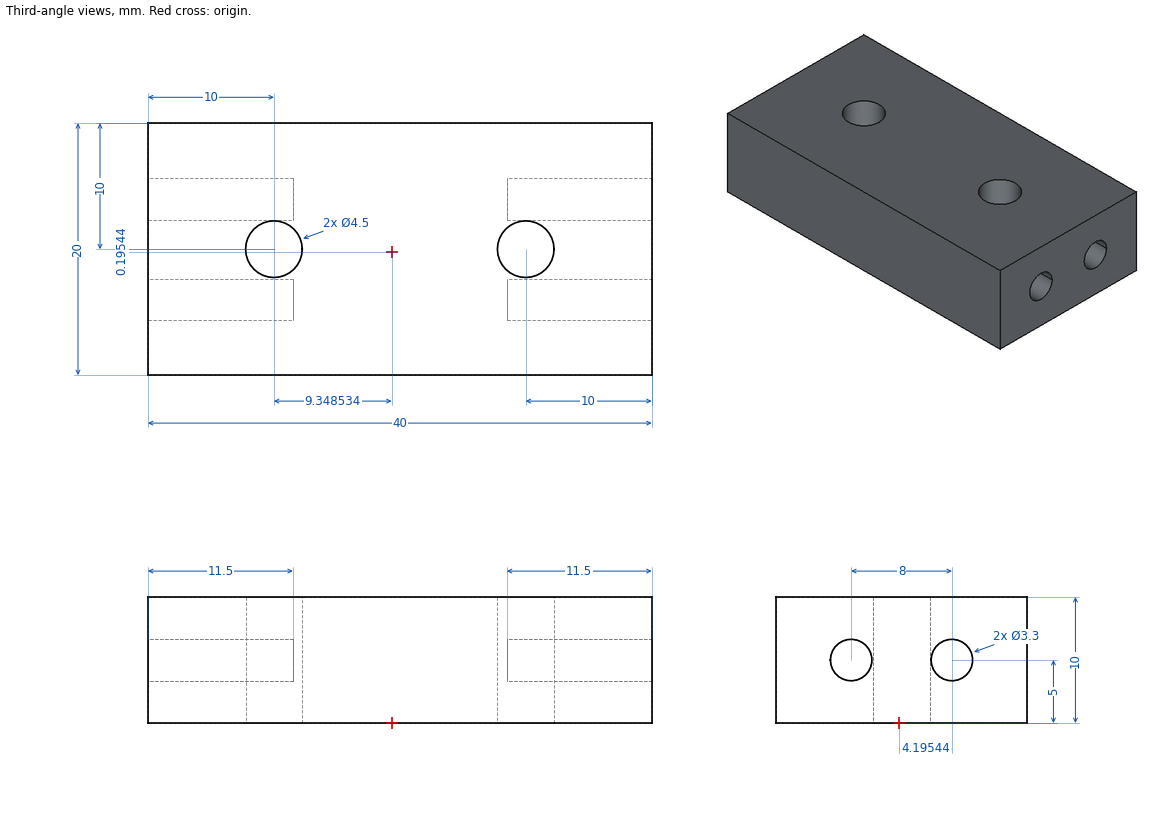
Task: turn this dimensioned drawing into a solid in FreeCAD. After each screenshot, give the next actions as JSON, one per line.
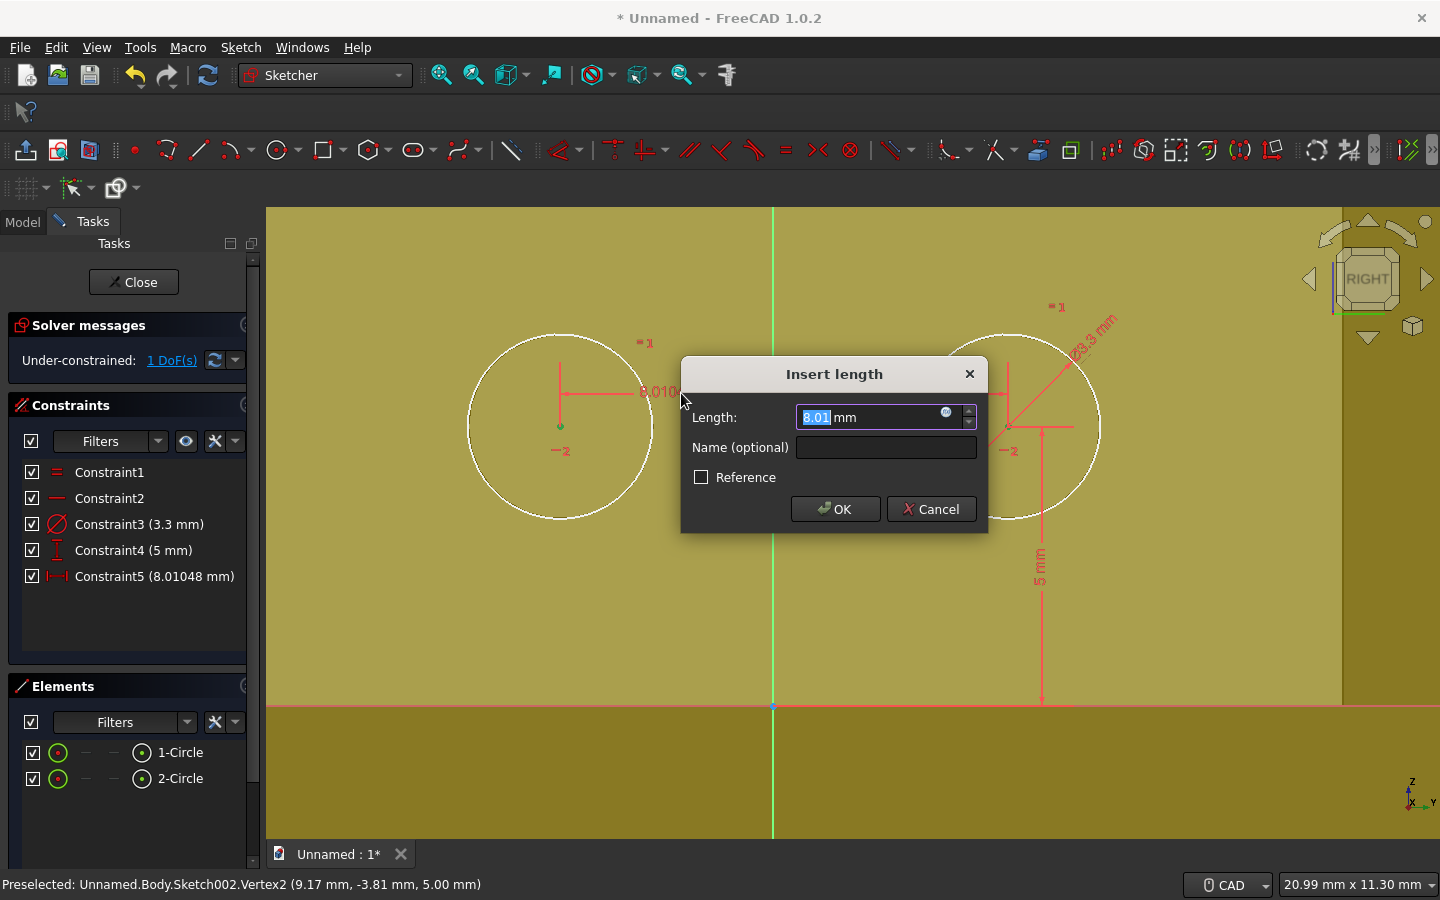
{"action": "type", "text": "8"}
{"action": "key", "text": "Return"}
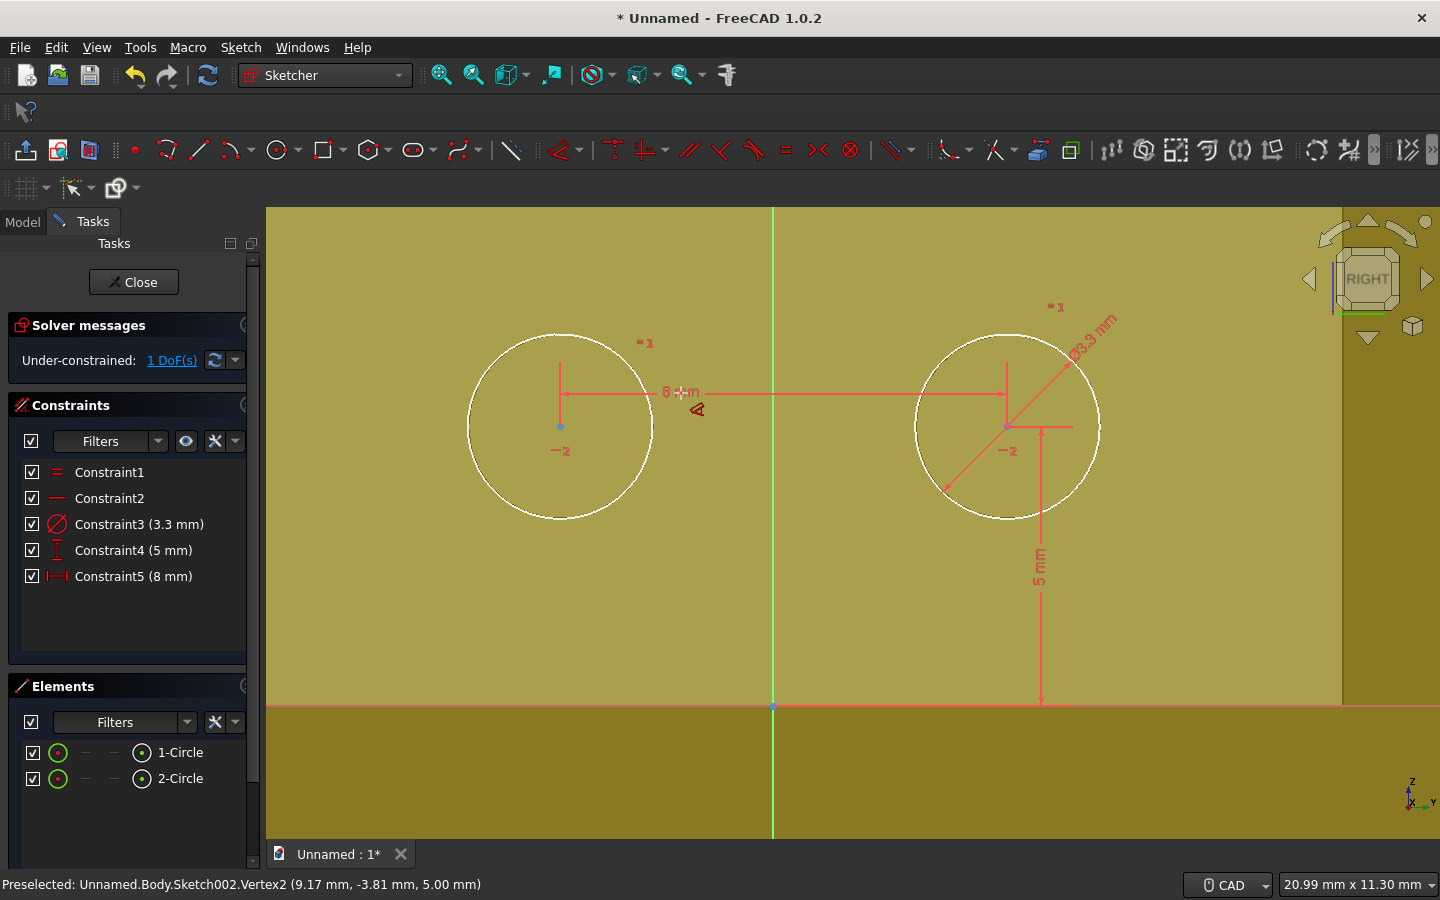
{"action": "left_click", "coordinate": [1007, 427]}
{"action": "left_click", "coordinate": [890, 740]}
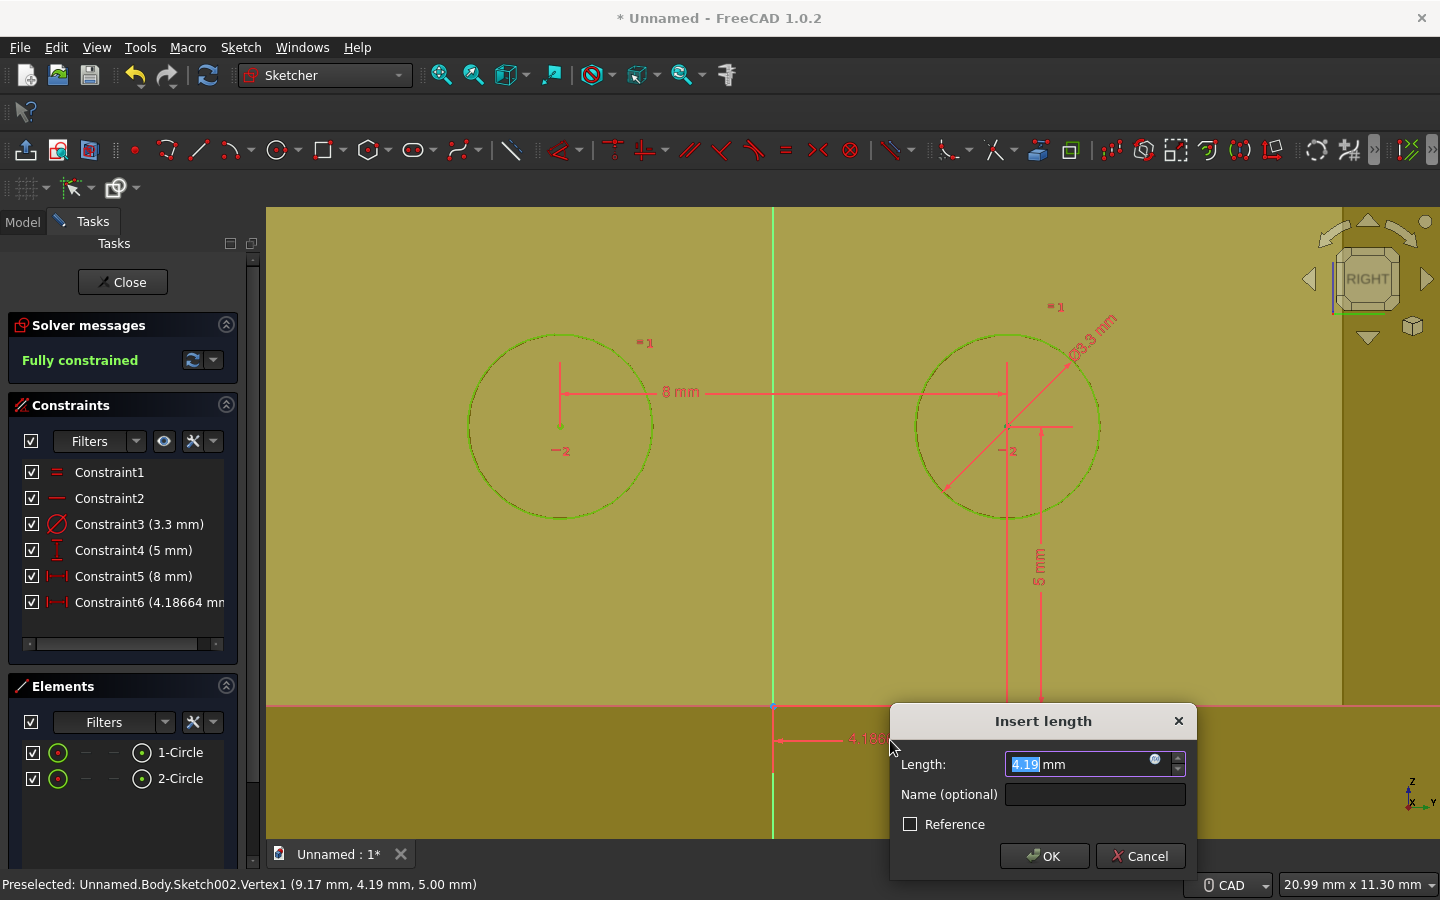
{"action": "type", "text": "4.19544"}
{"action": "key", "text": "Return"}
{"action": "key", "text": "Escape"}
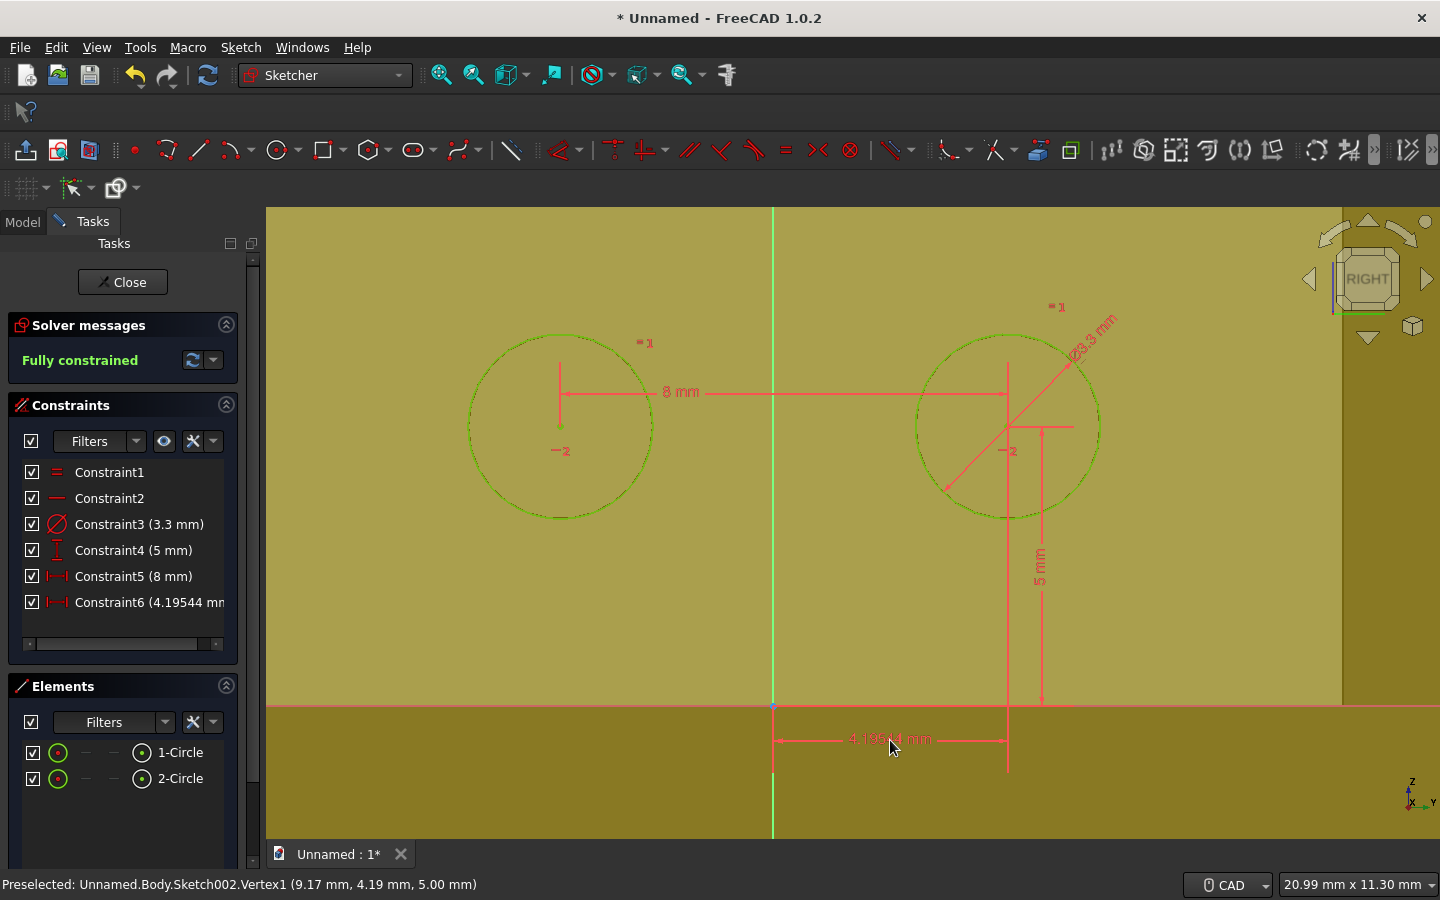
{"action": "left_click", "coordinate": [123, 282]}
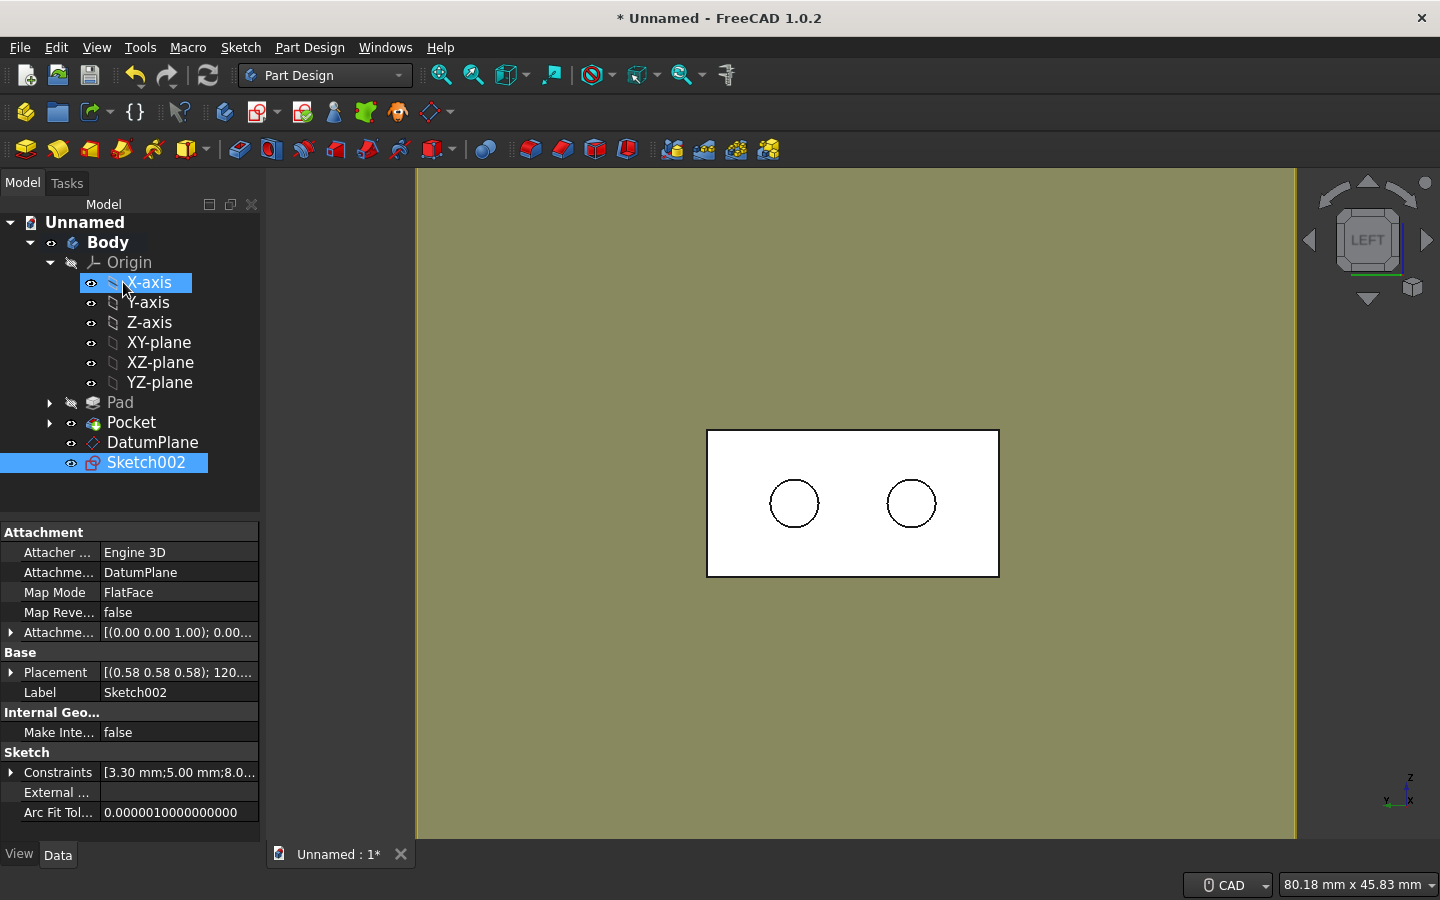
{"action": "left_click", "coordinate": [240, 150]}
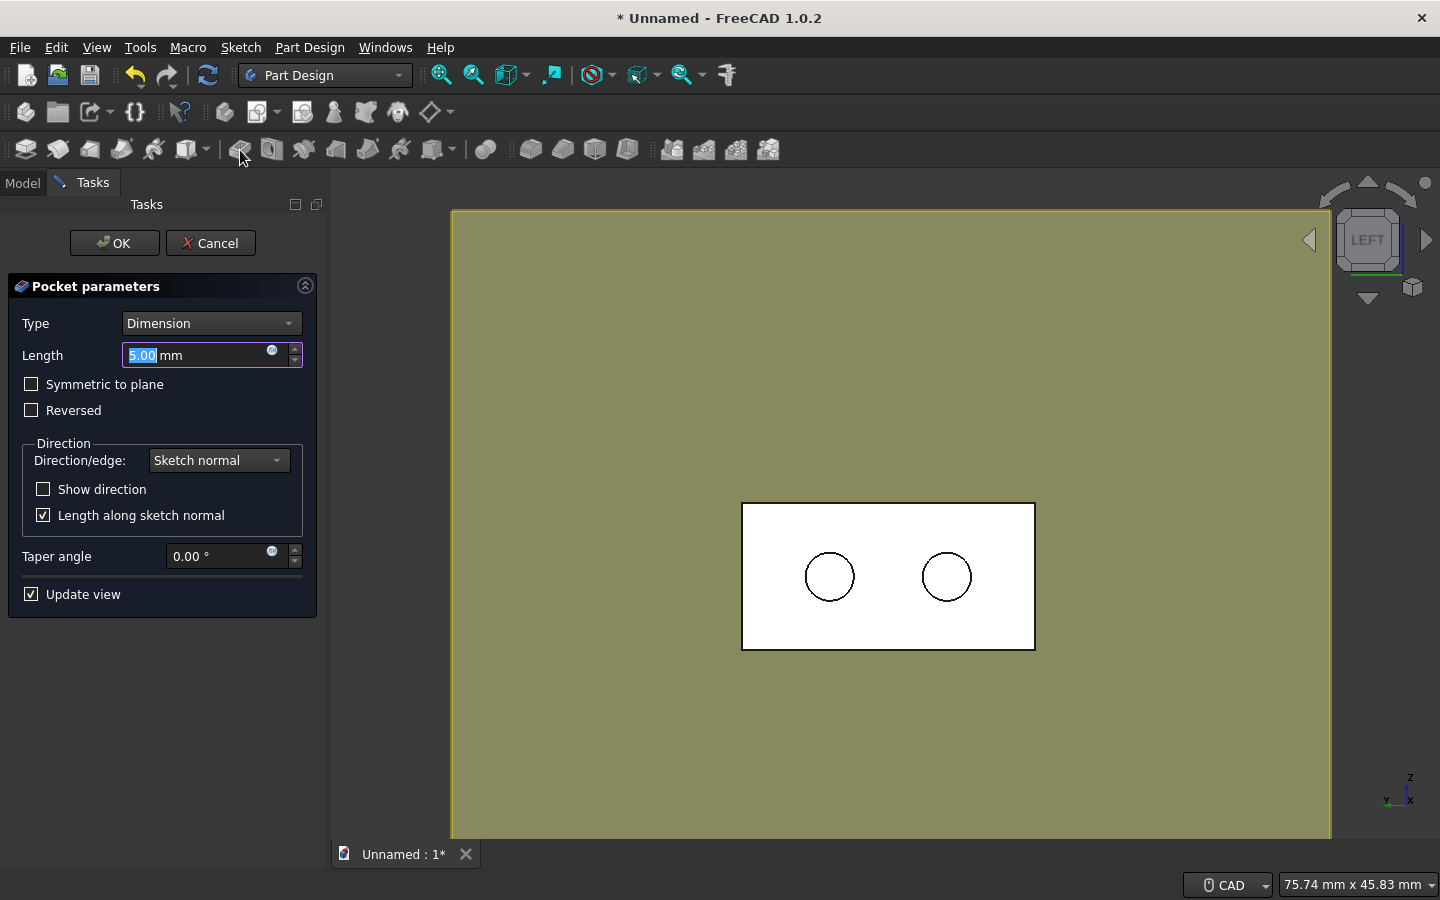
{"action": "type", "text": "11.5"}
{"action": "key", "text": "Tab"}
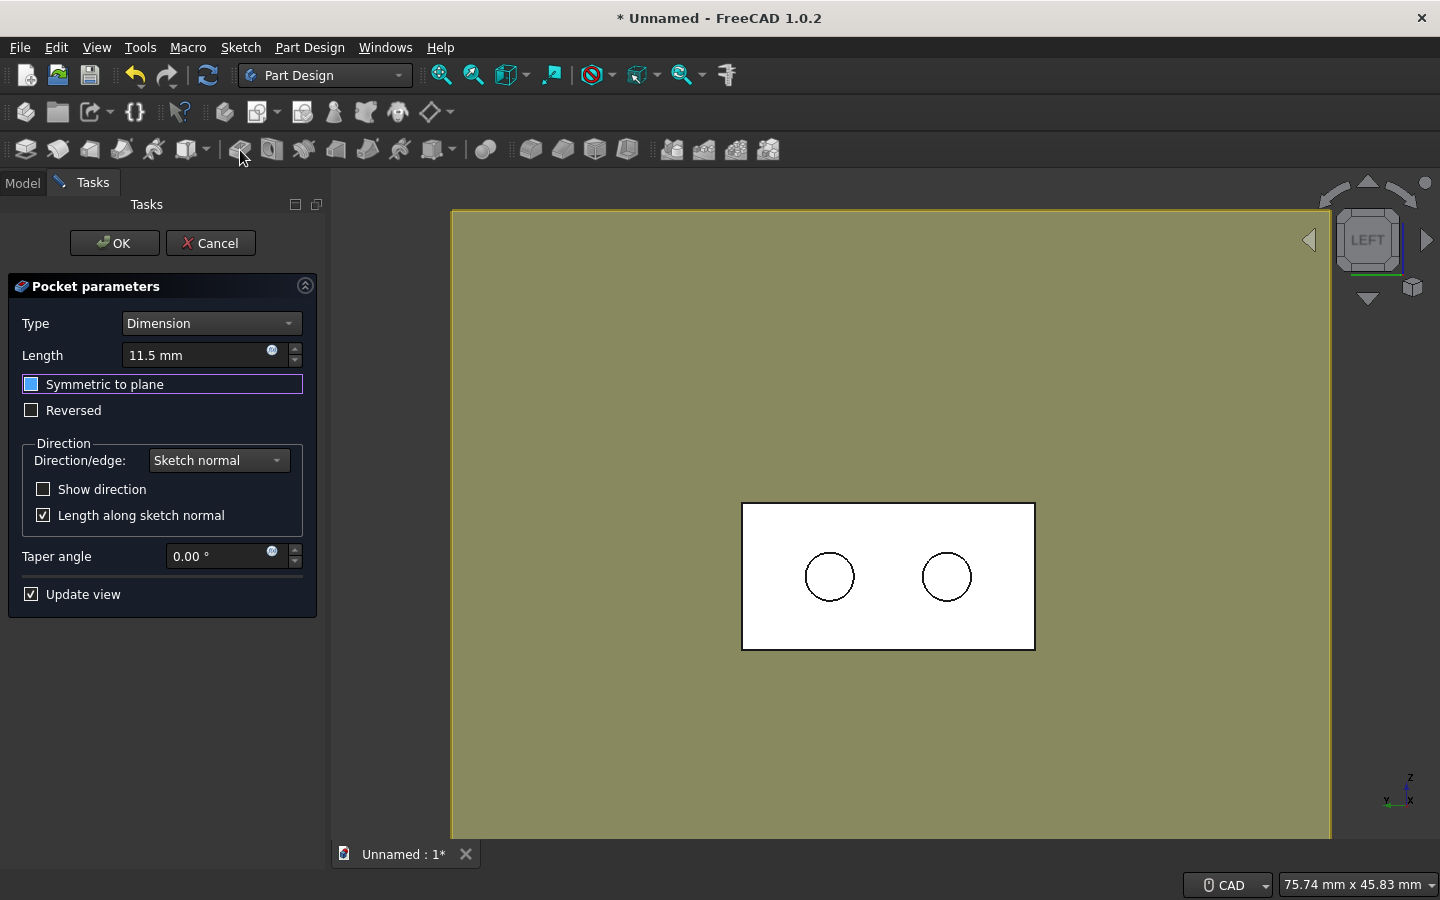
{"action": "left_click", "coordinate": [30, 410]}